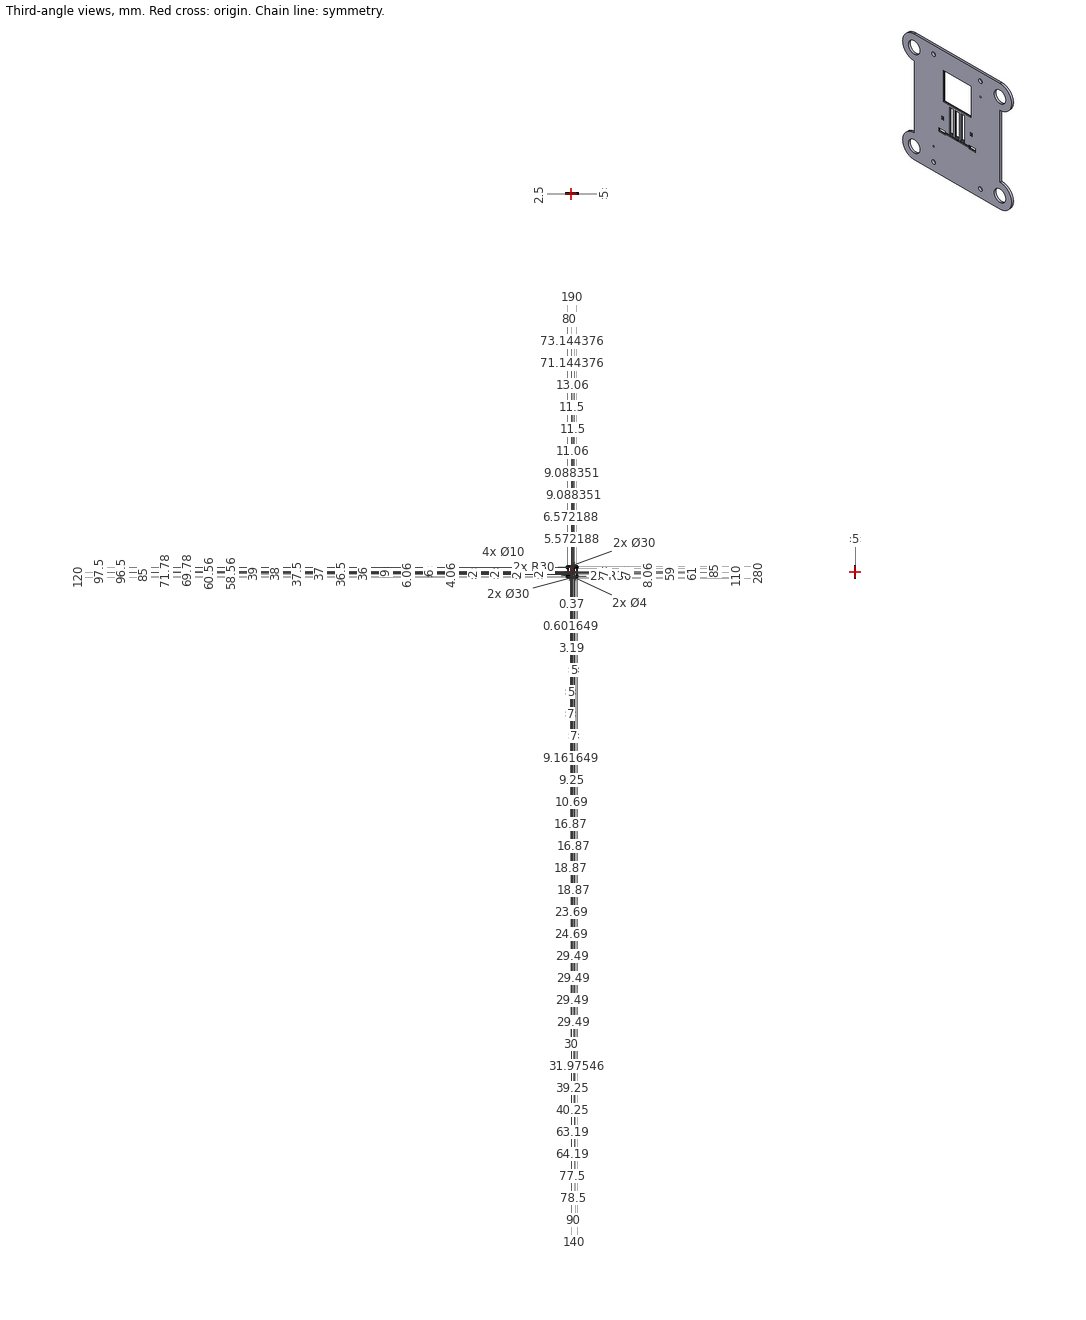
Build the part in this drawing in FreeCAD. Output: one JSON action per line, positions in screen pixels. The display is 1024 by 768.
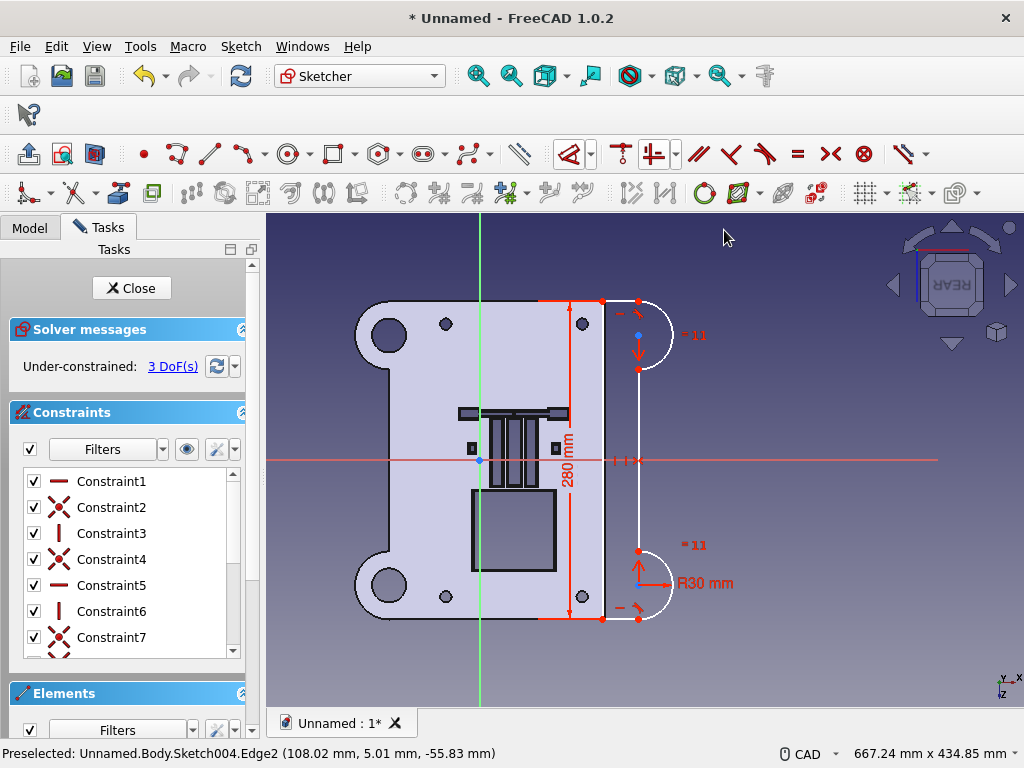
{"action": "left_click", "coordinate": [639, 301]}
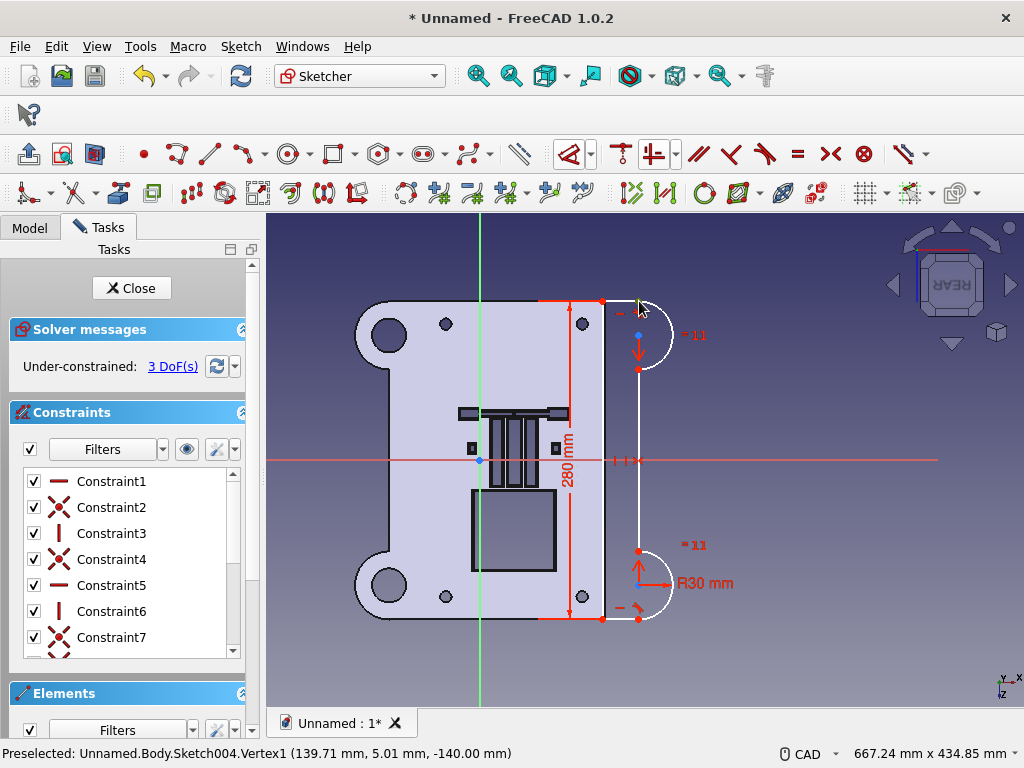
{"action": "key", "text": "l"}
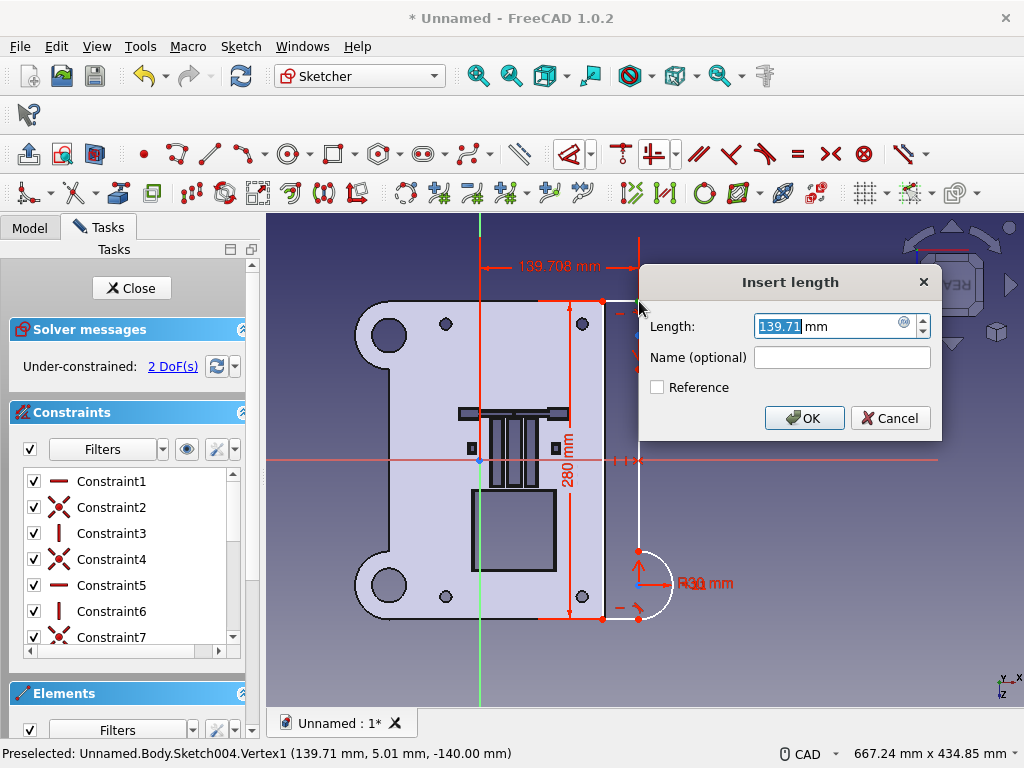
{"action": "type", "text": "140"}
{"action": "key", "text": "Return"}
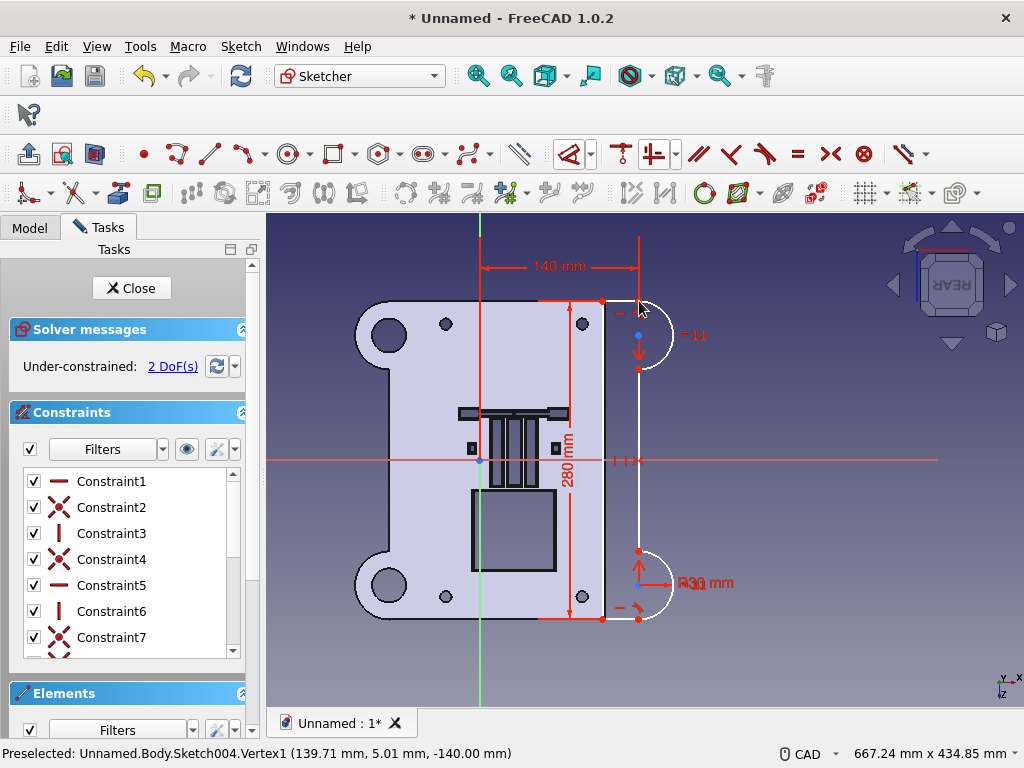
{"action": "left_click", "coordinate": [639, 551]}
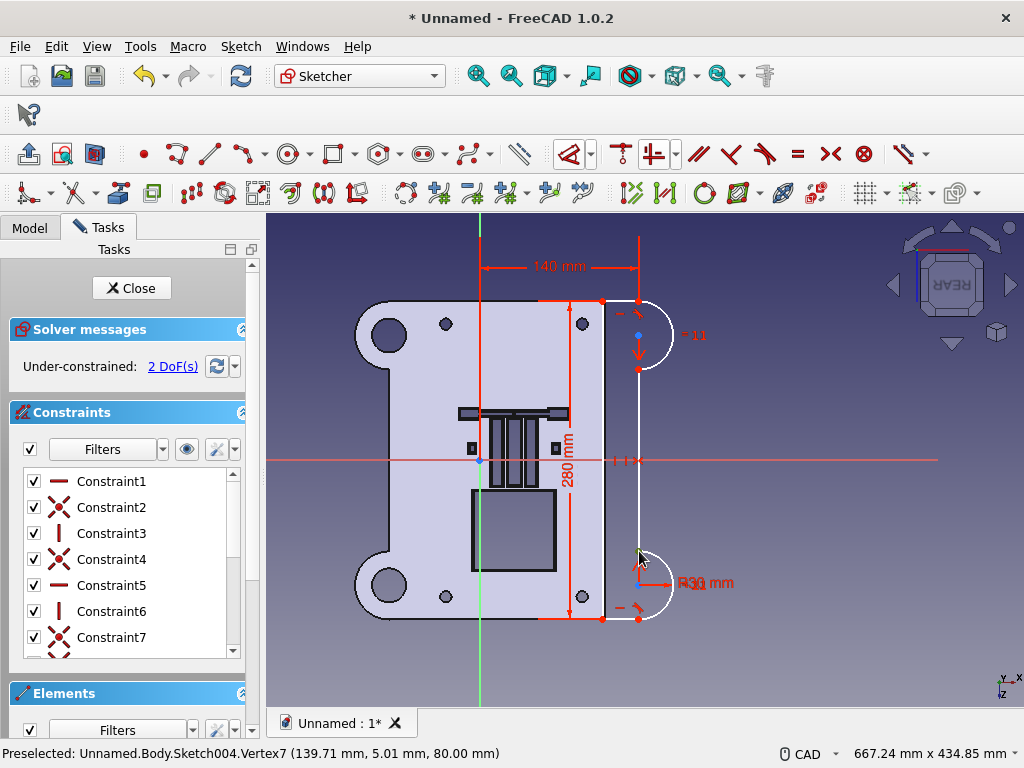
{"action": "left_click", "coordinate": [590, 154]}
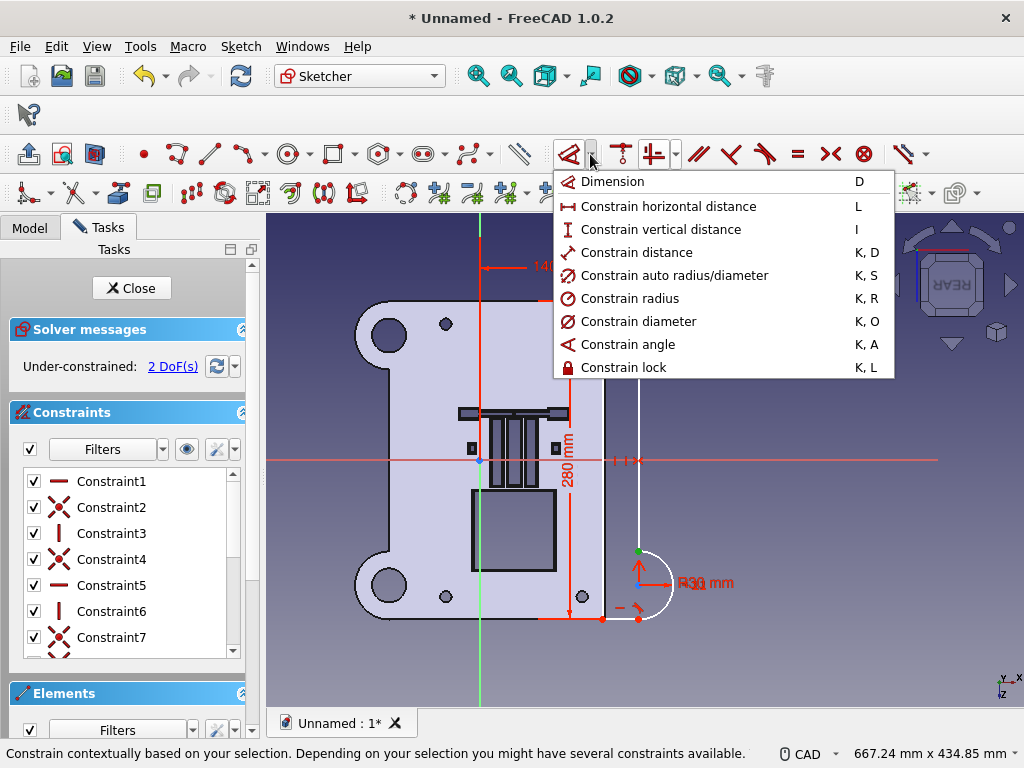
{"action": "left_click", "coordinate": [724, 206]}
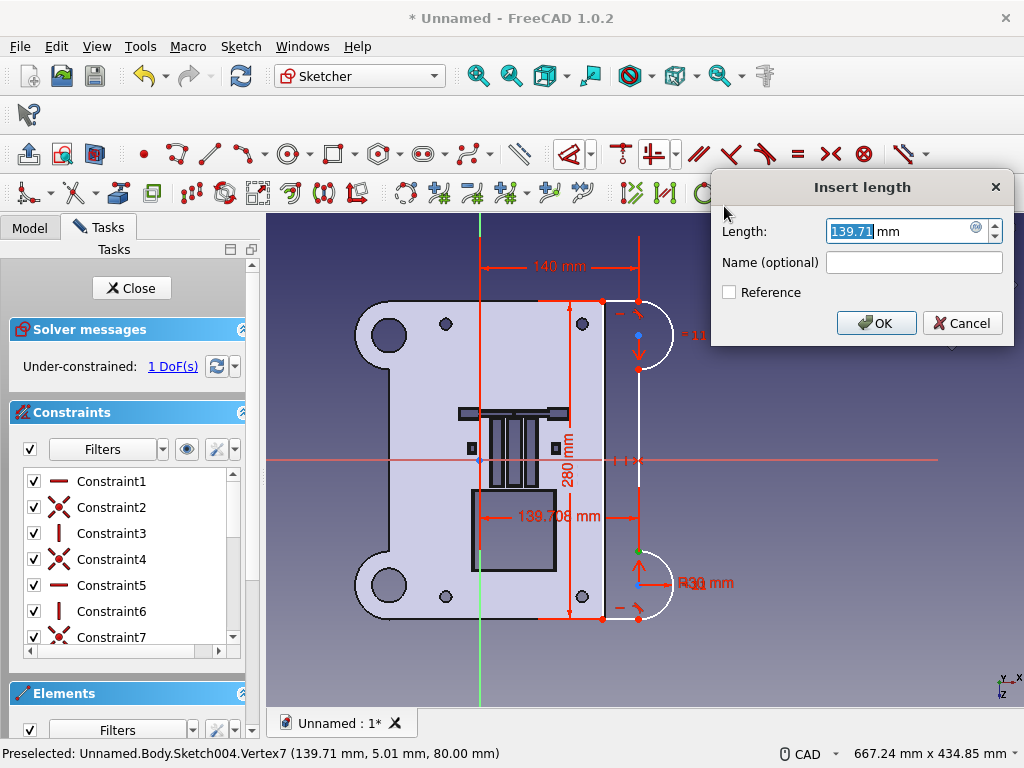
{"action": "type", "text": "140"}
{"action": "key", "text": "Return"}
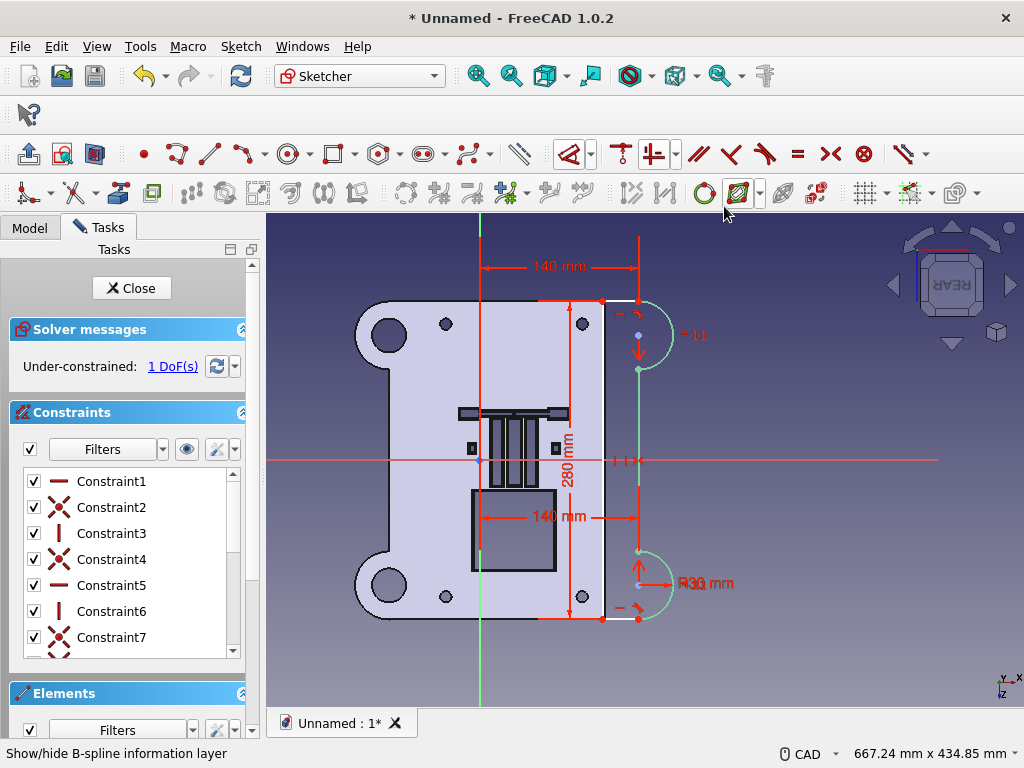
{"action": "scroll", "coordinate": [628, 301], "scroll_direction": "up", "scroll_amount": 2}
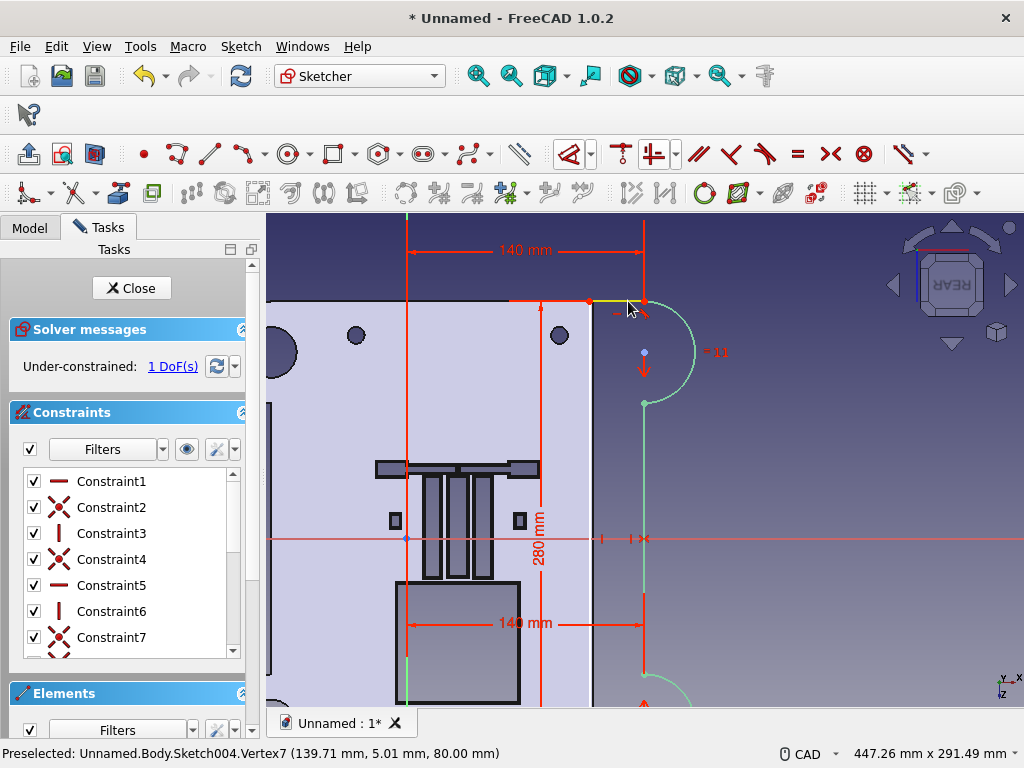
{"action": "left_click", "coordinate": [628, 301]}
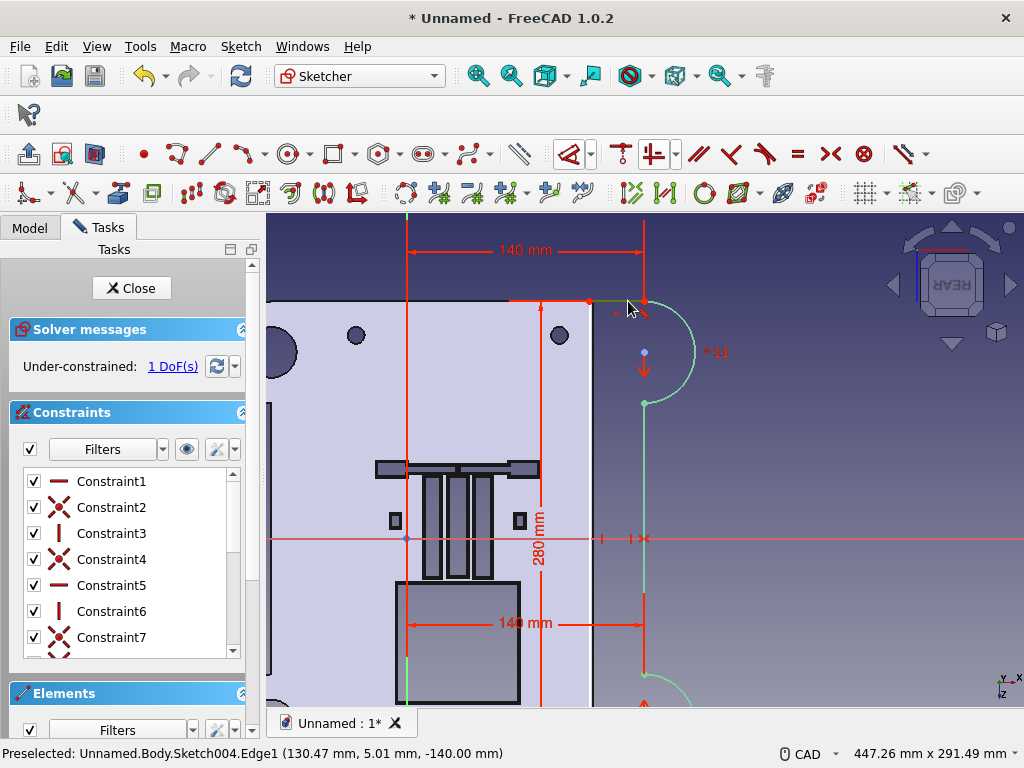
{"action": "left_click", "coordinate": [590, 154]}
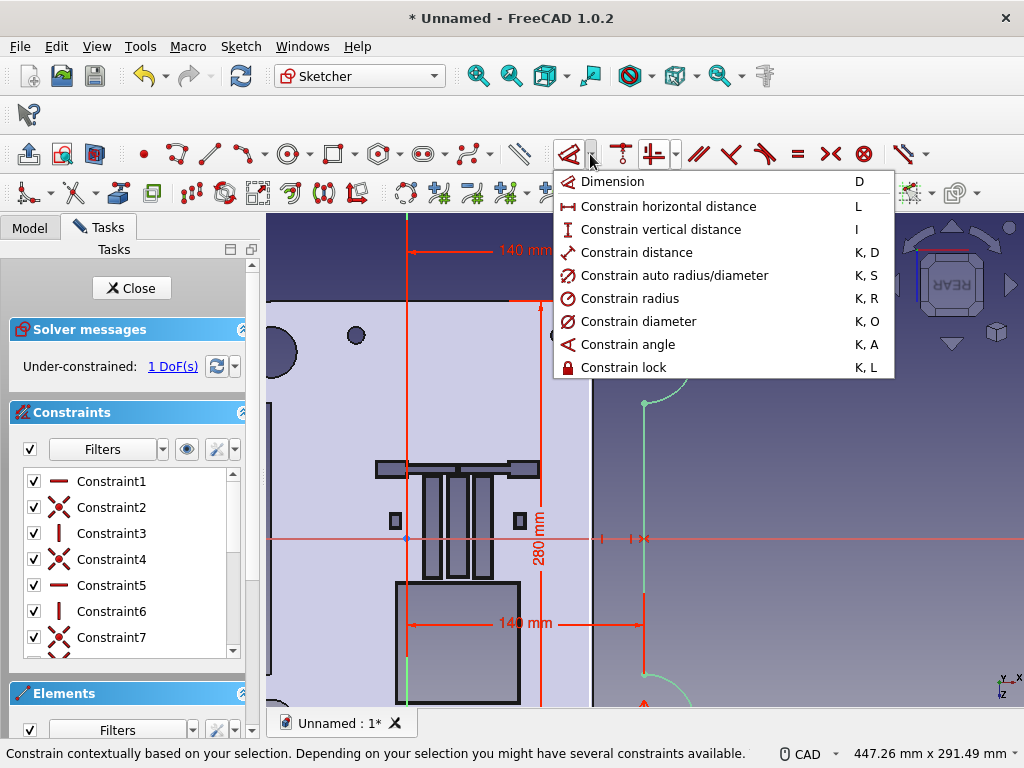
{"action": "left_click", "coordinate": [724, 206]}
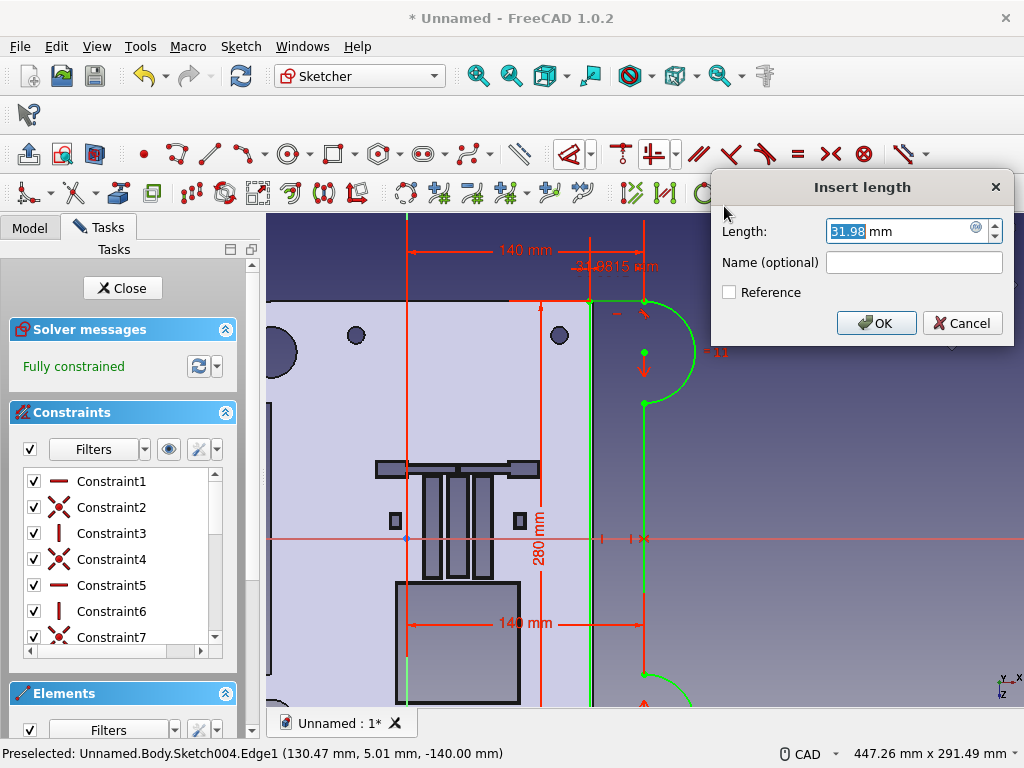
{"action": "type", "text": "31.97546"}
{"action": "key", "text": "Return"}